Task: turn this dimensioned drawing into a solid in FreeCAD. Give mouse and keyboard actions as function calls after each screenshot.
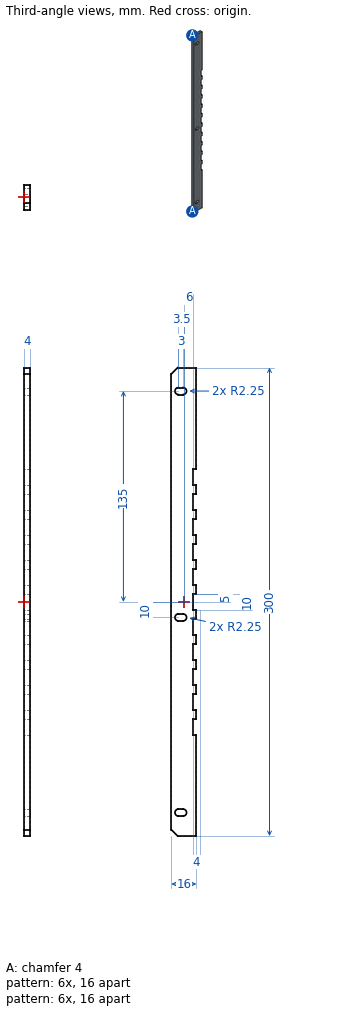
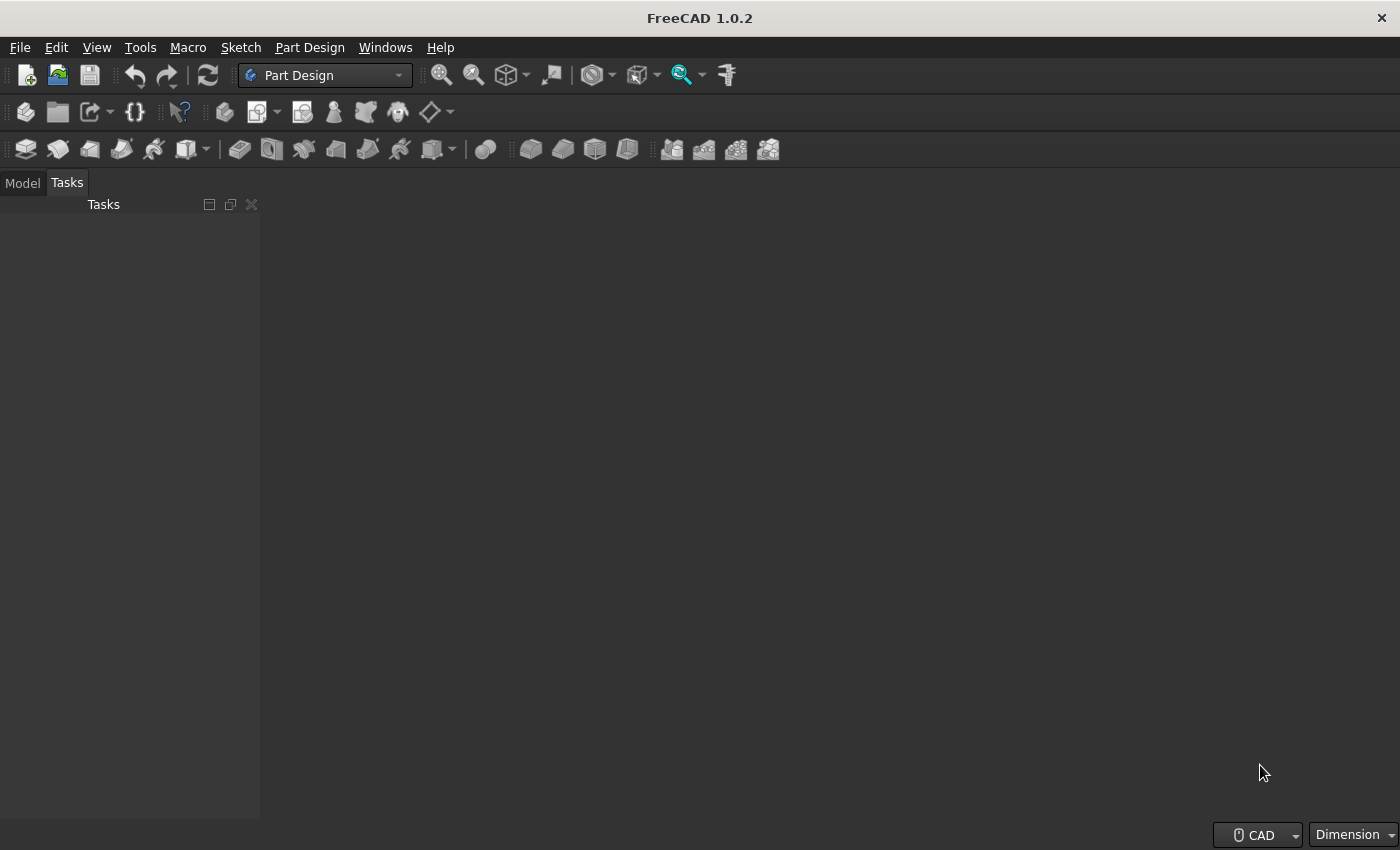
key(ctrl+n)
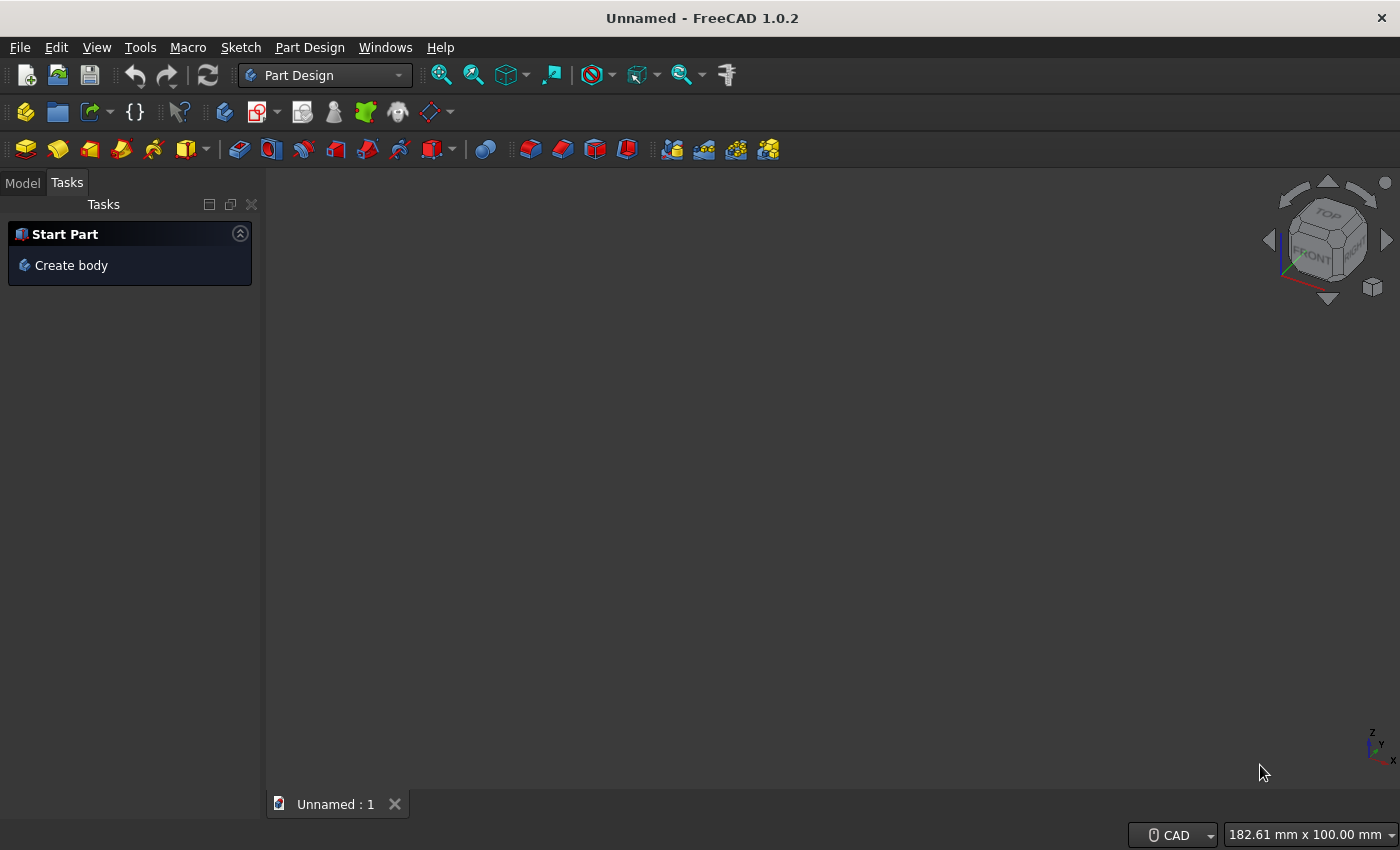
click(258, 112)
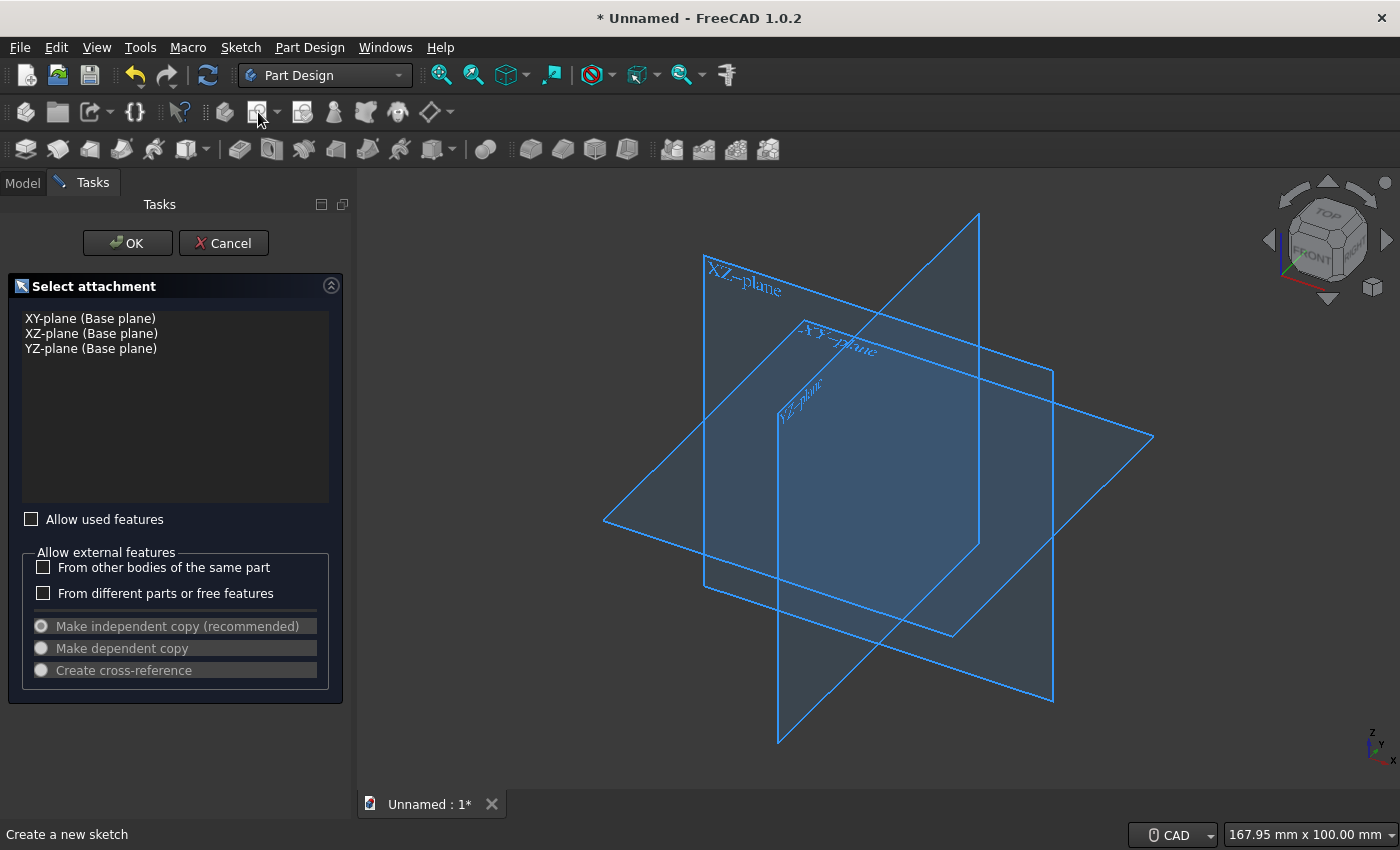
click(82, 348)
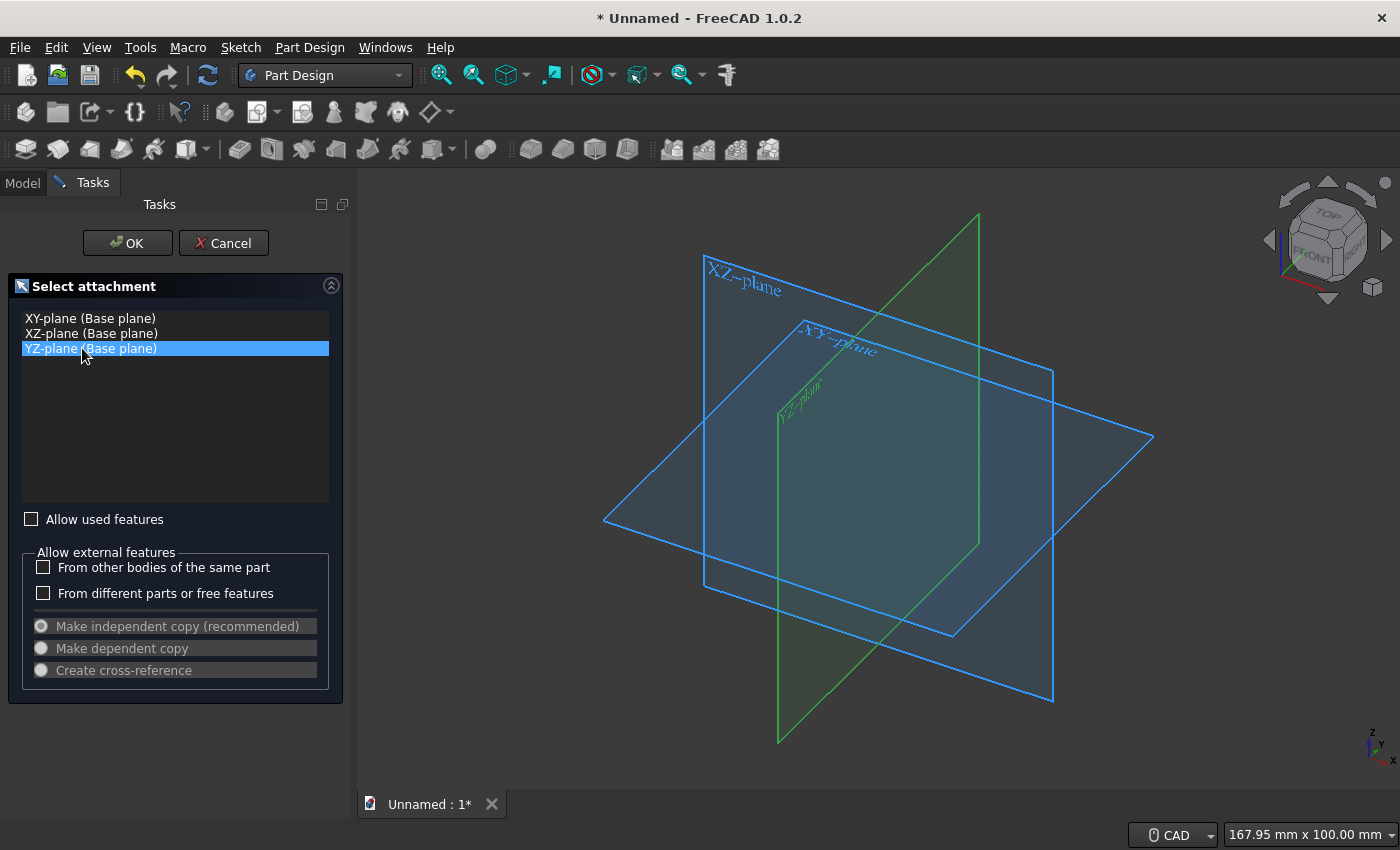
click(128, 243)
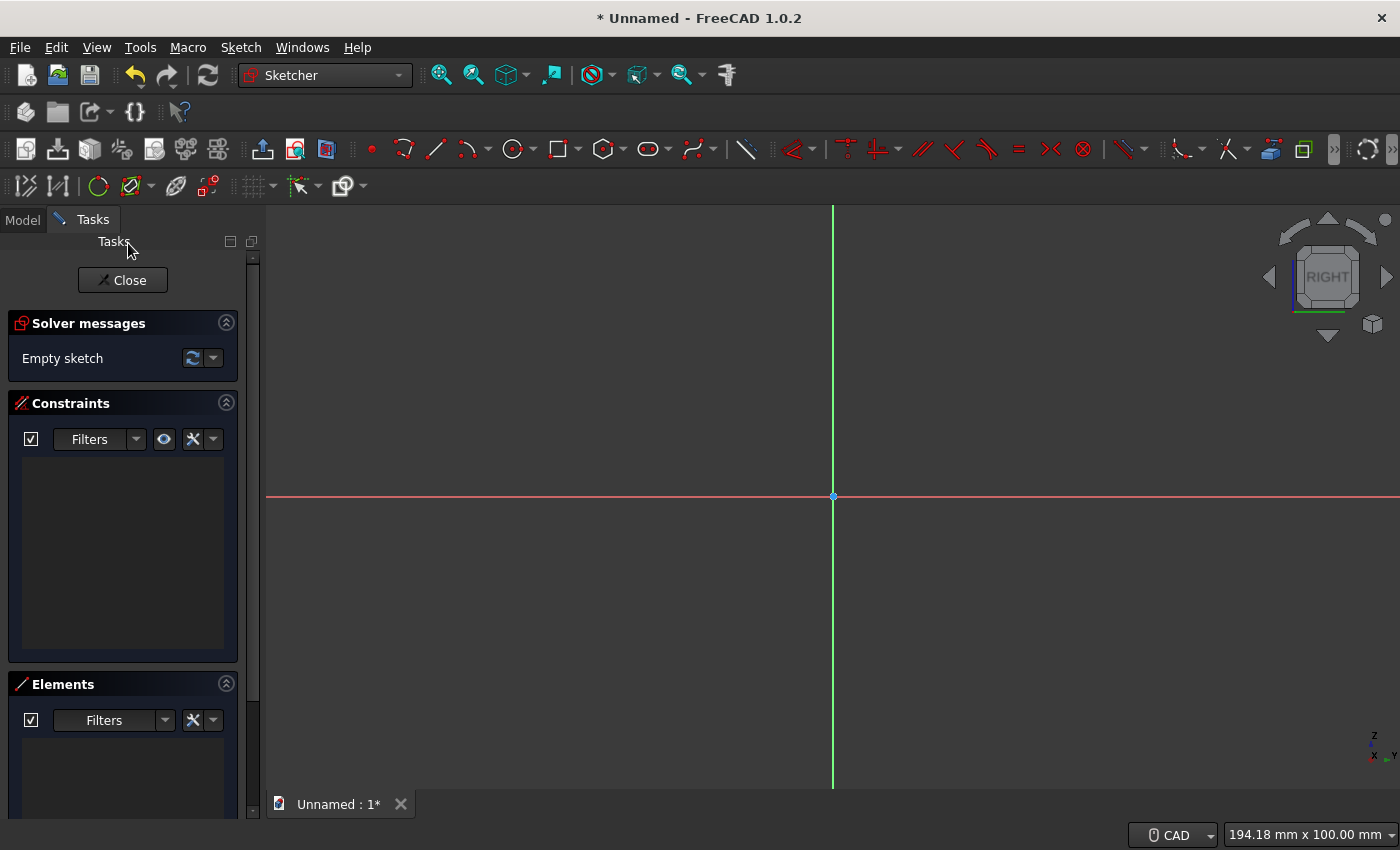
scroll(747, 497, down, 8)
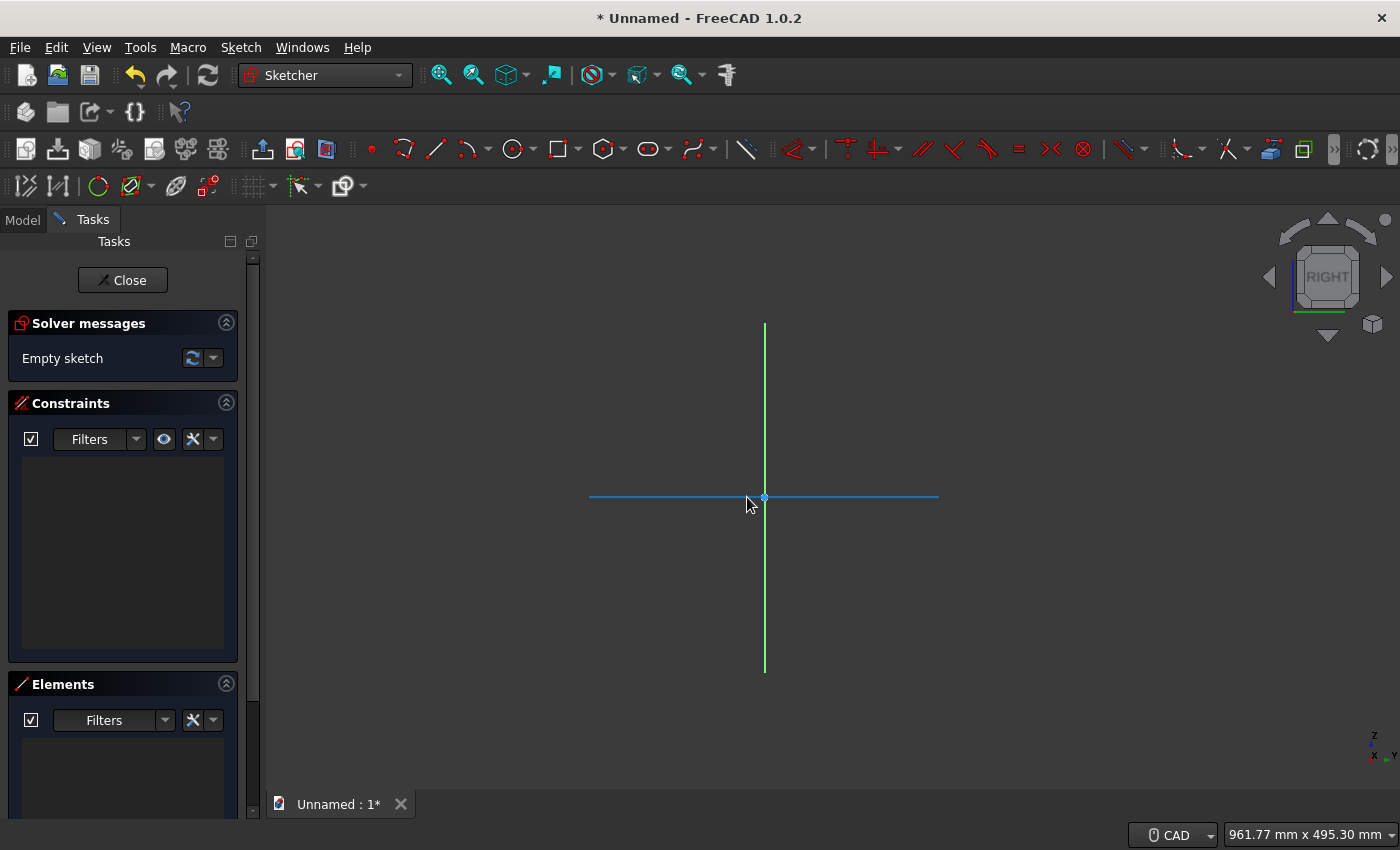
key(g)
key(v)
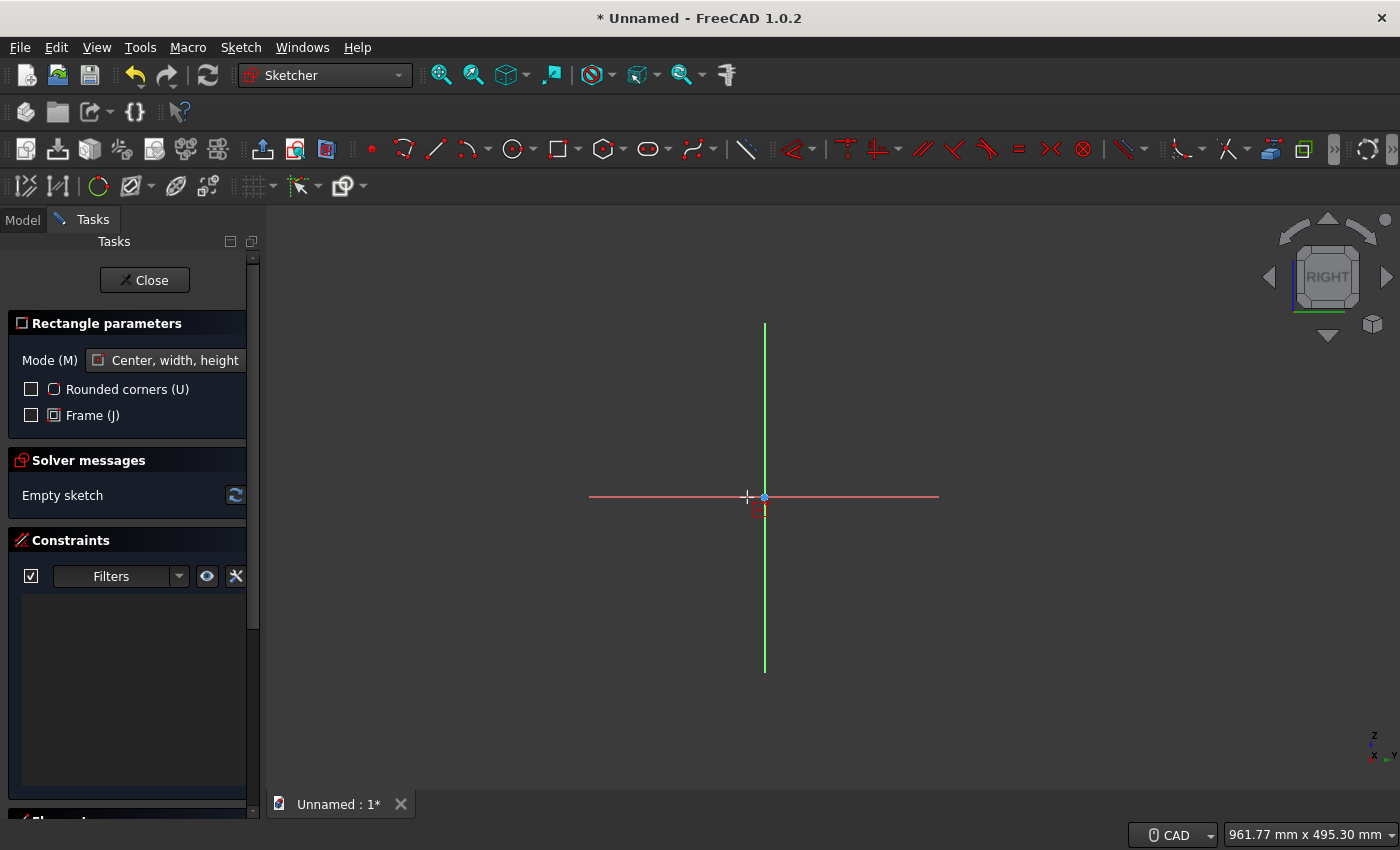
scroll(765, 497, up, 3)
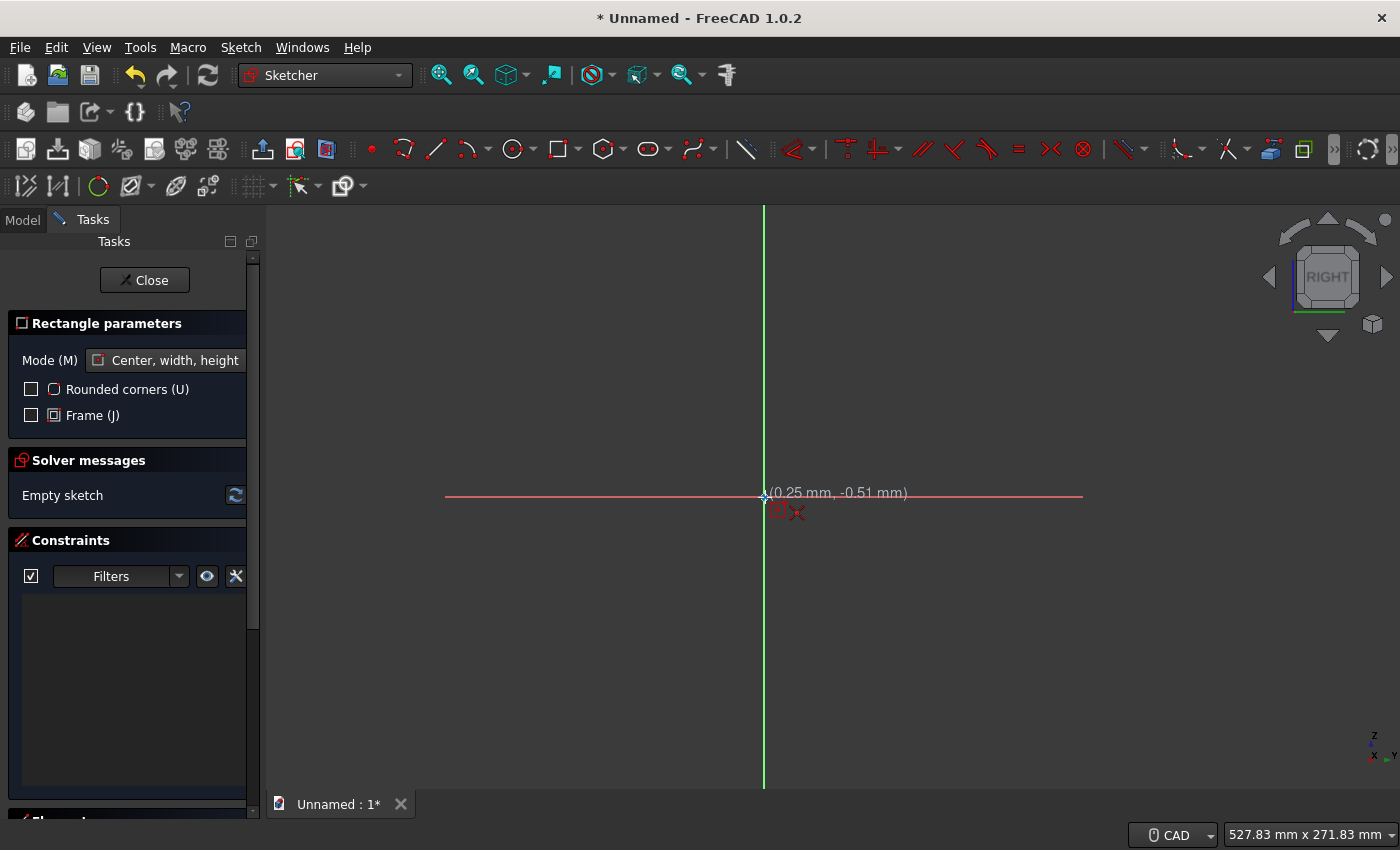
click(764, 497)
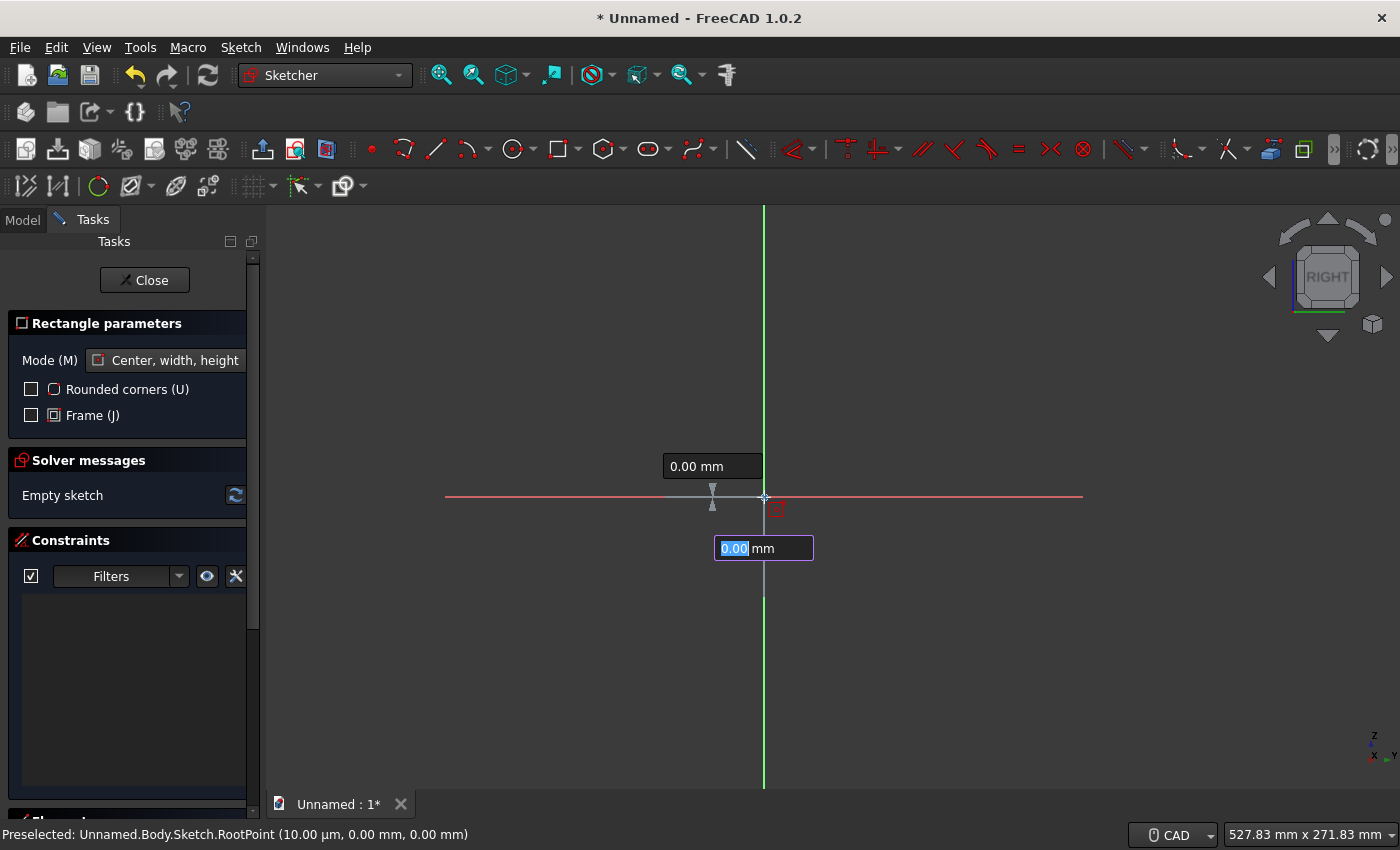
scroll(765, 497, down, 3)